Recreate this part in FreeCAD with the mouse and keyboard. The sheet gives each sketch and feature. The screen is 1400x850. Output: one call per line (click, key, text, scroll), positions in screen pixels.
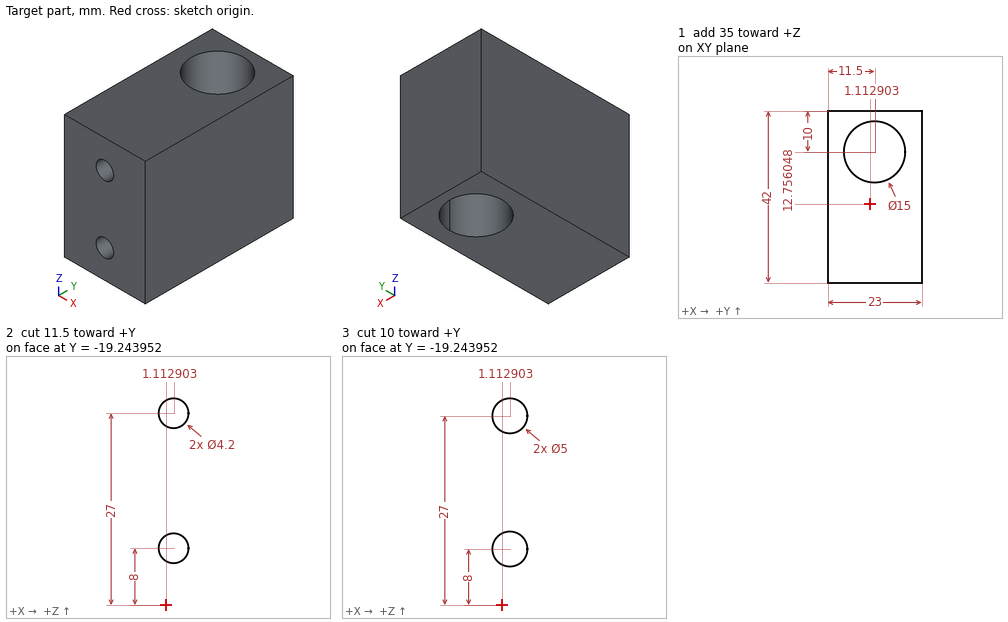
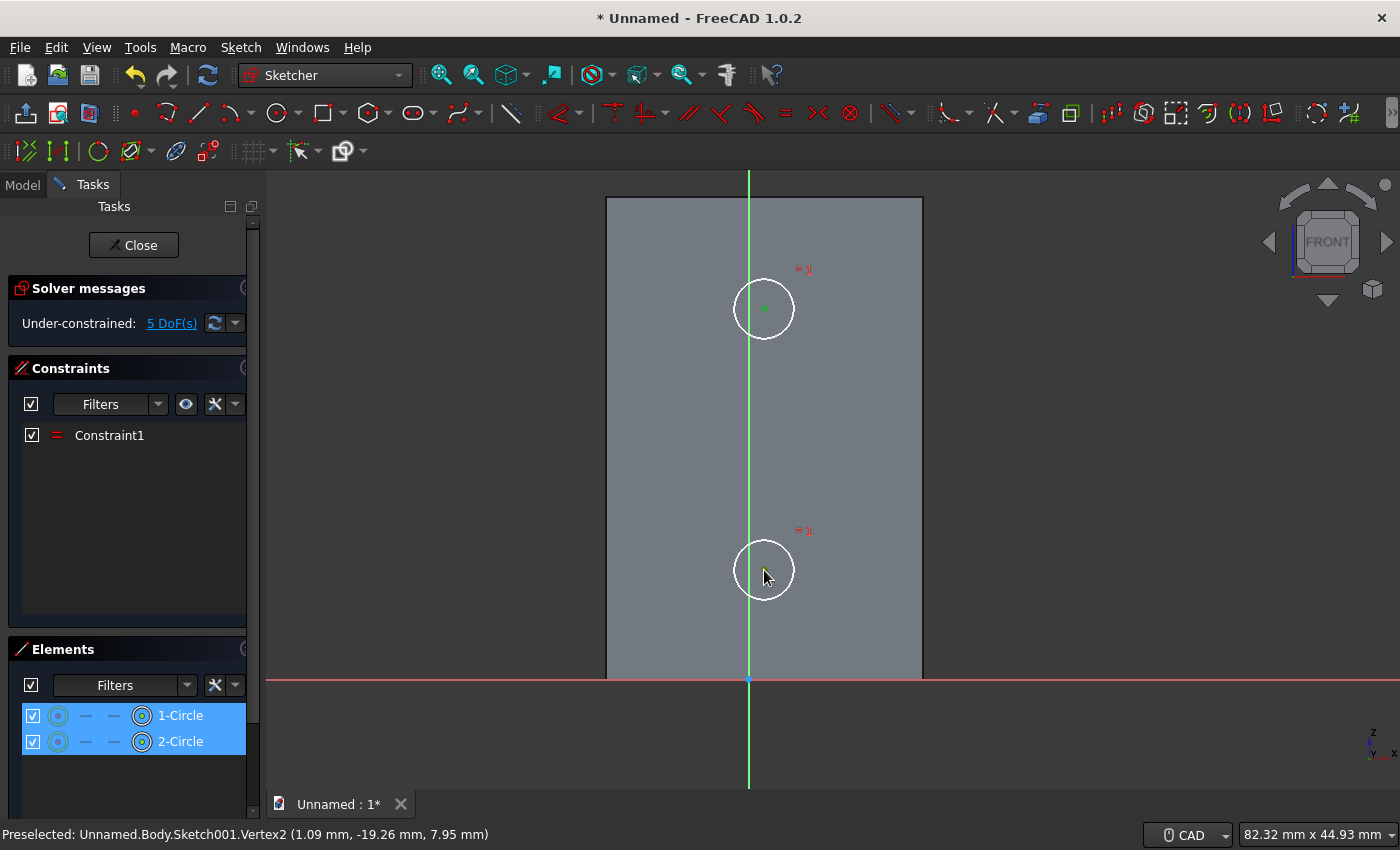
key(v)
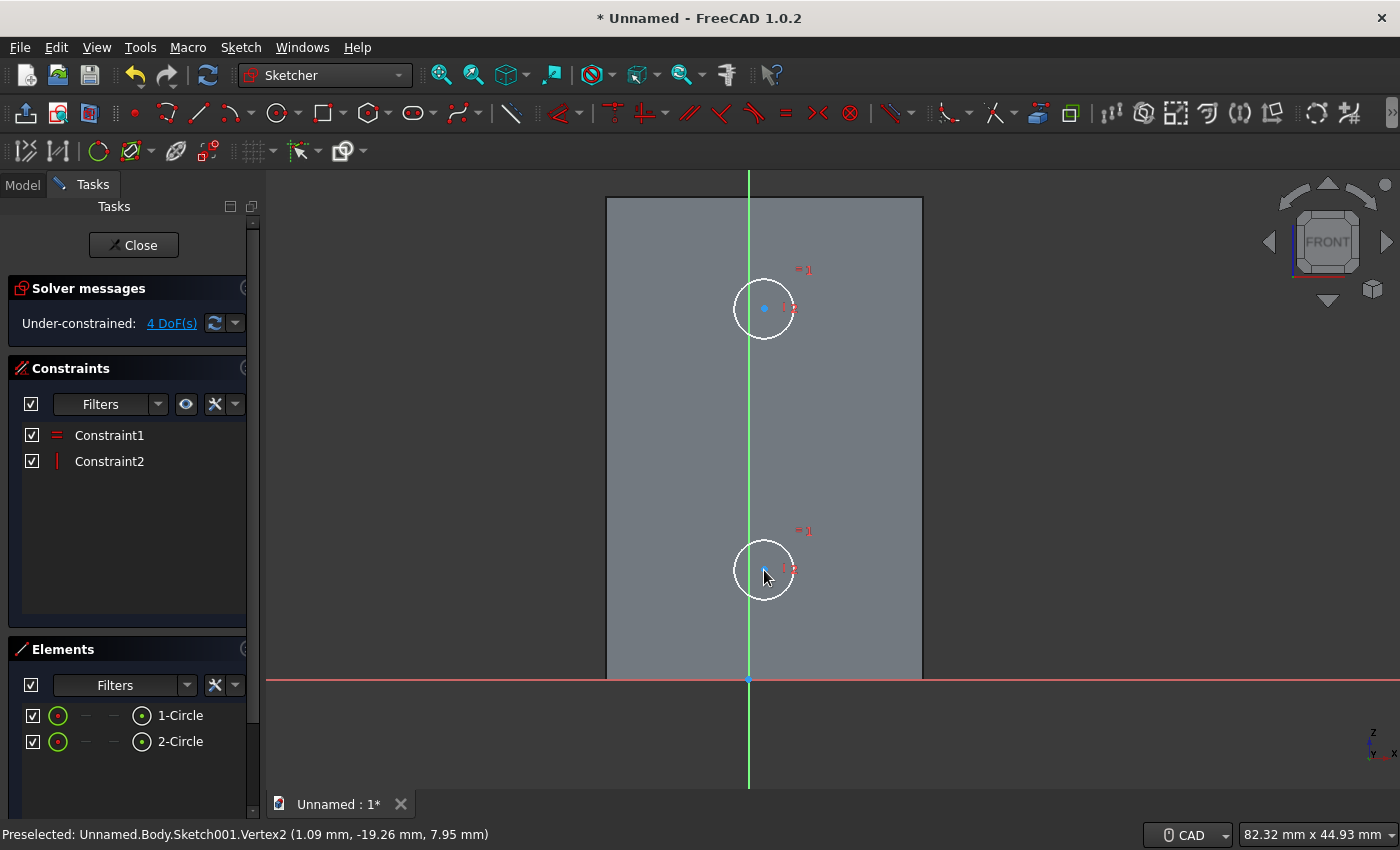
click(558, 114)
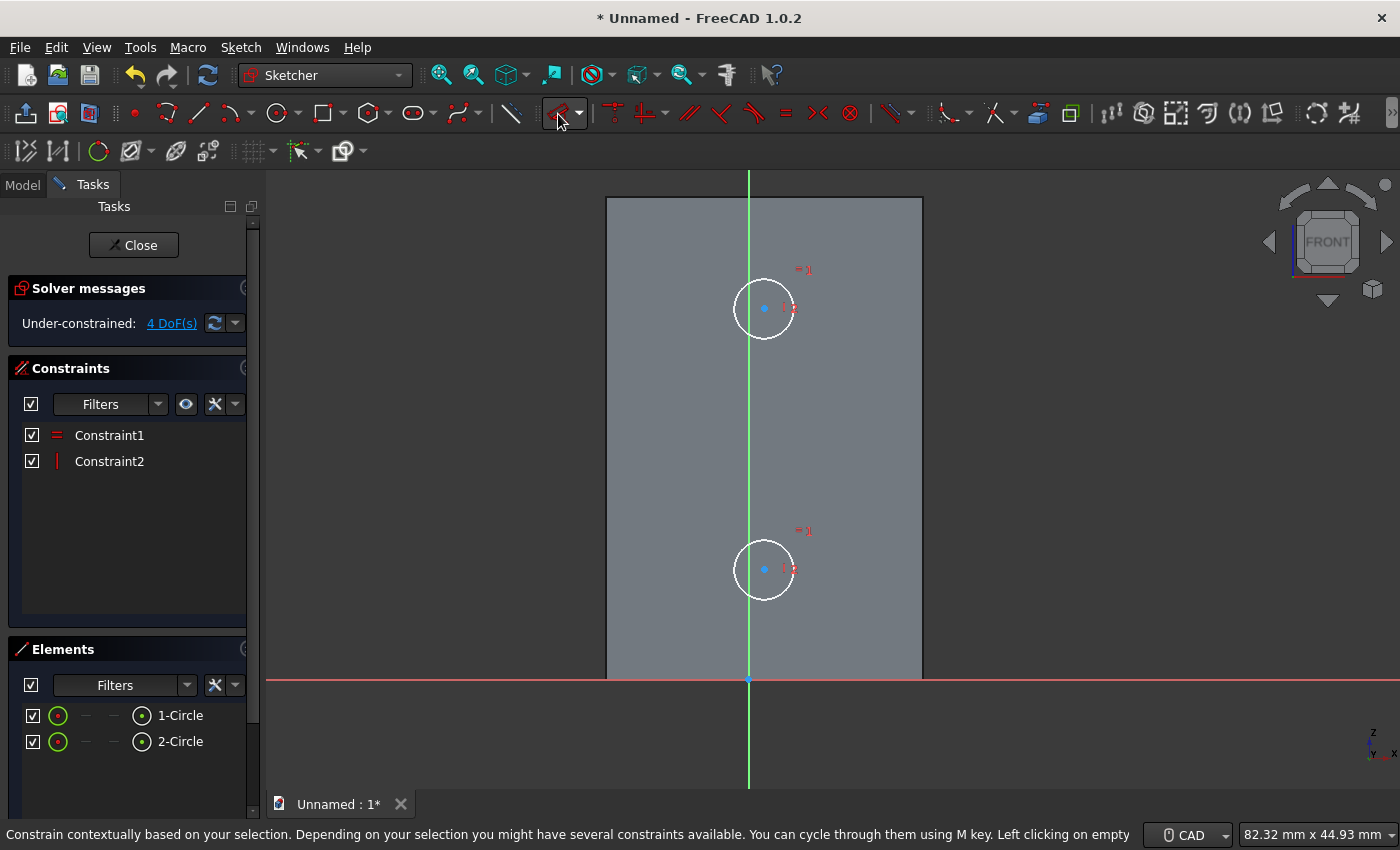
click(785, 288)
click(808, 265)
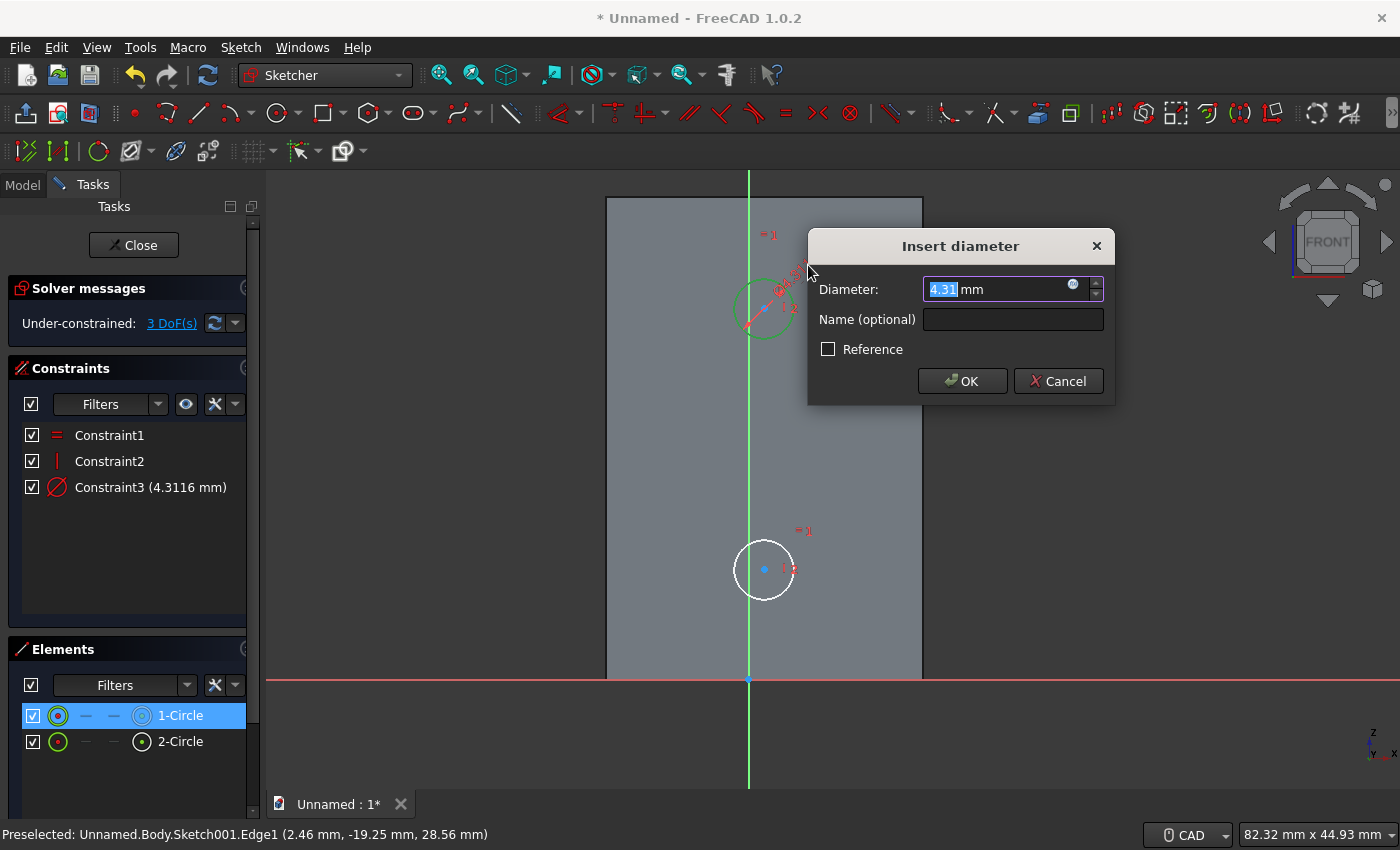
text(4.2)
key(Return)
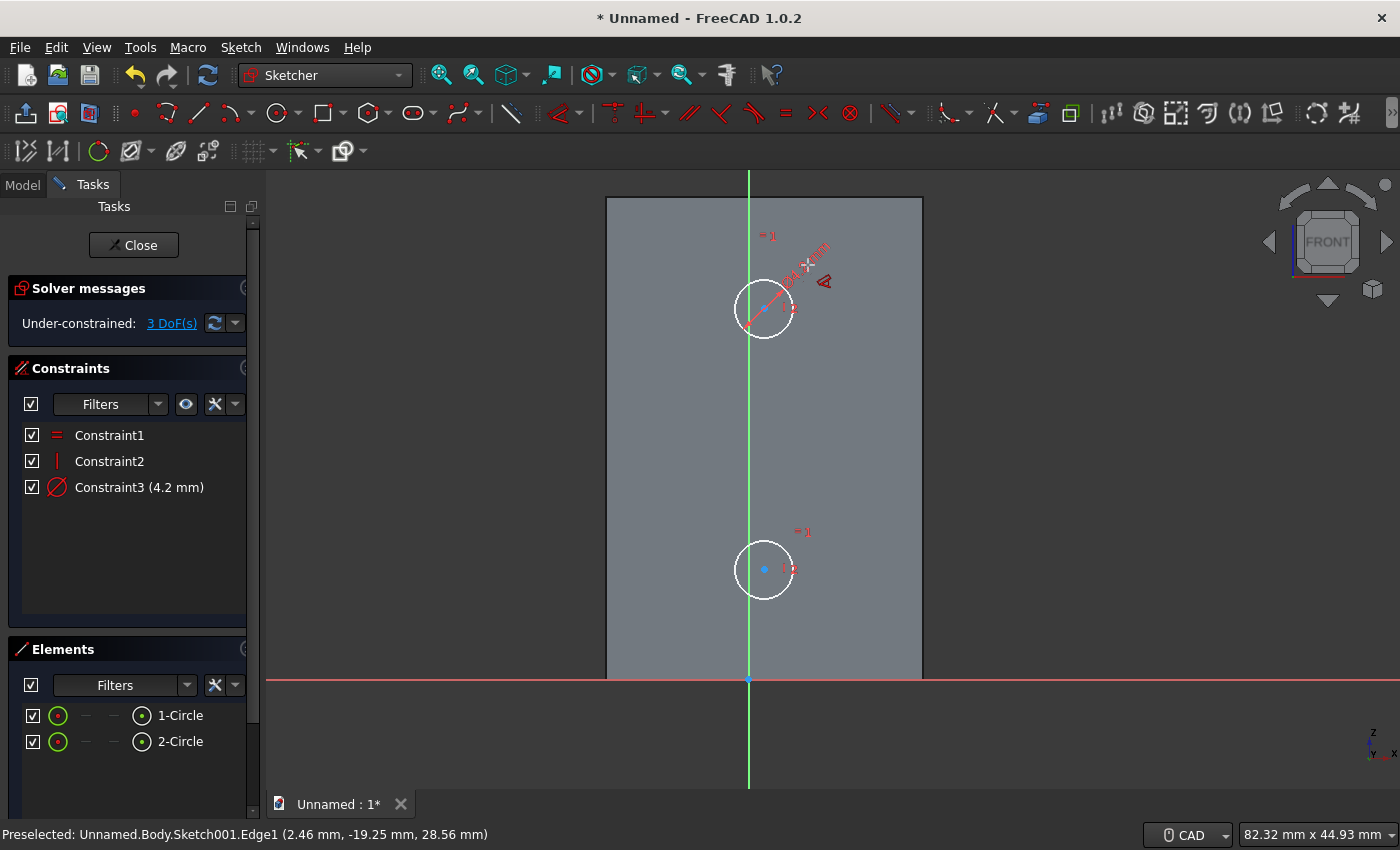
click(764, 570)
click(715, 625)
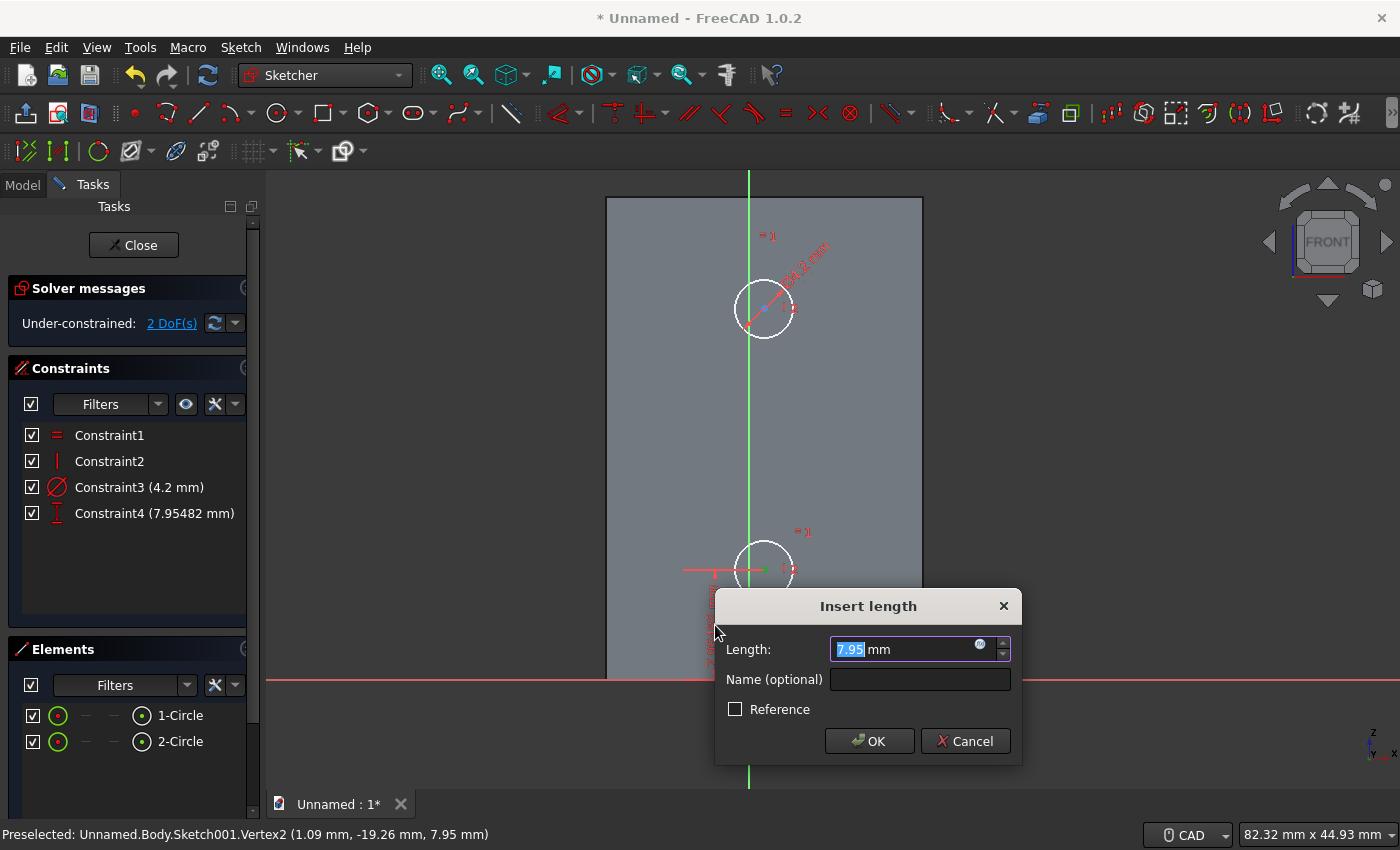
text(8)
key(Return)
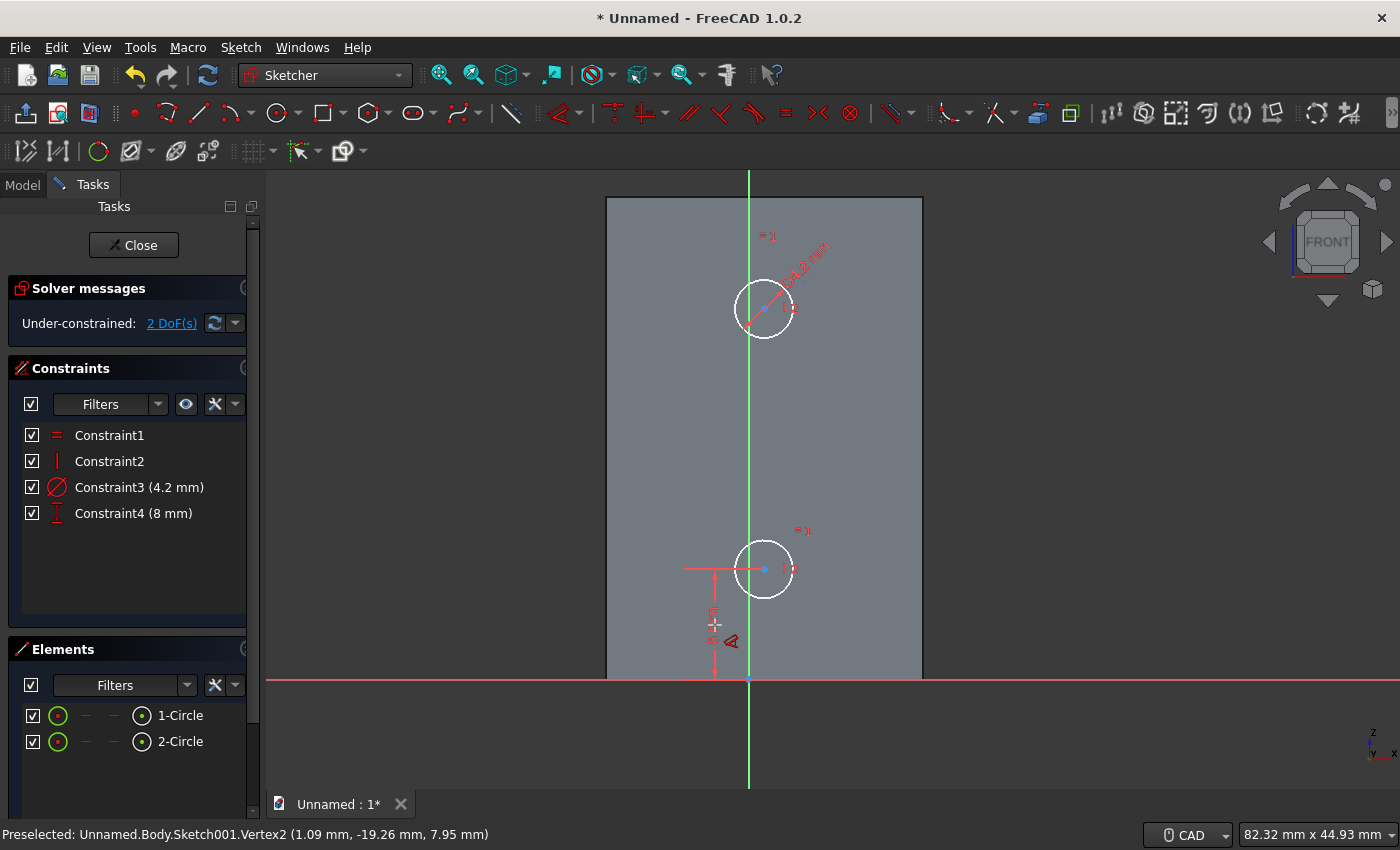
click(764, 309)
click(715, 494)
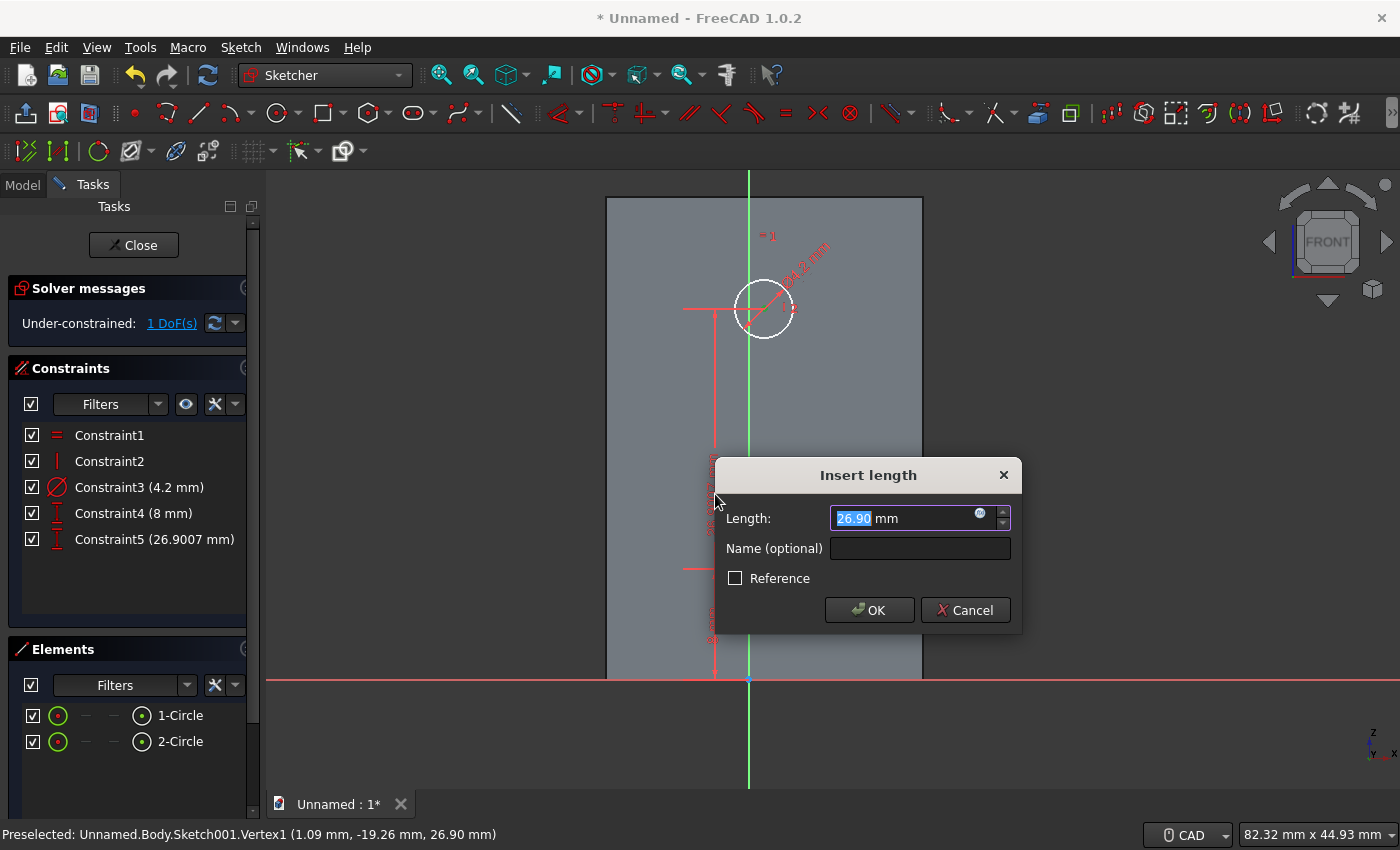
text(27)
key(Return)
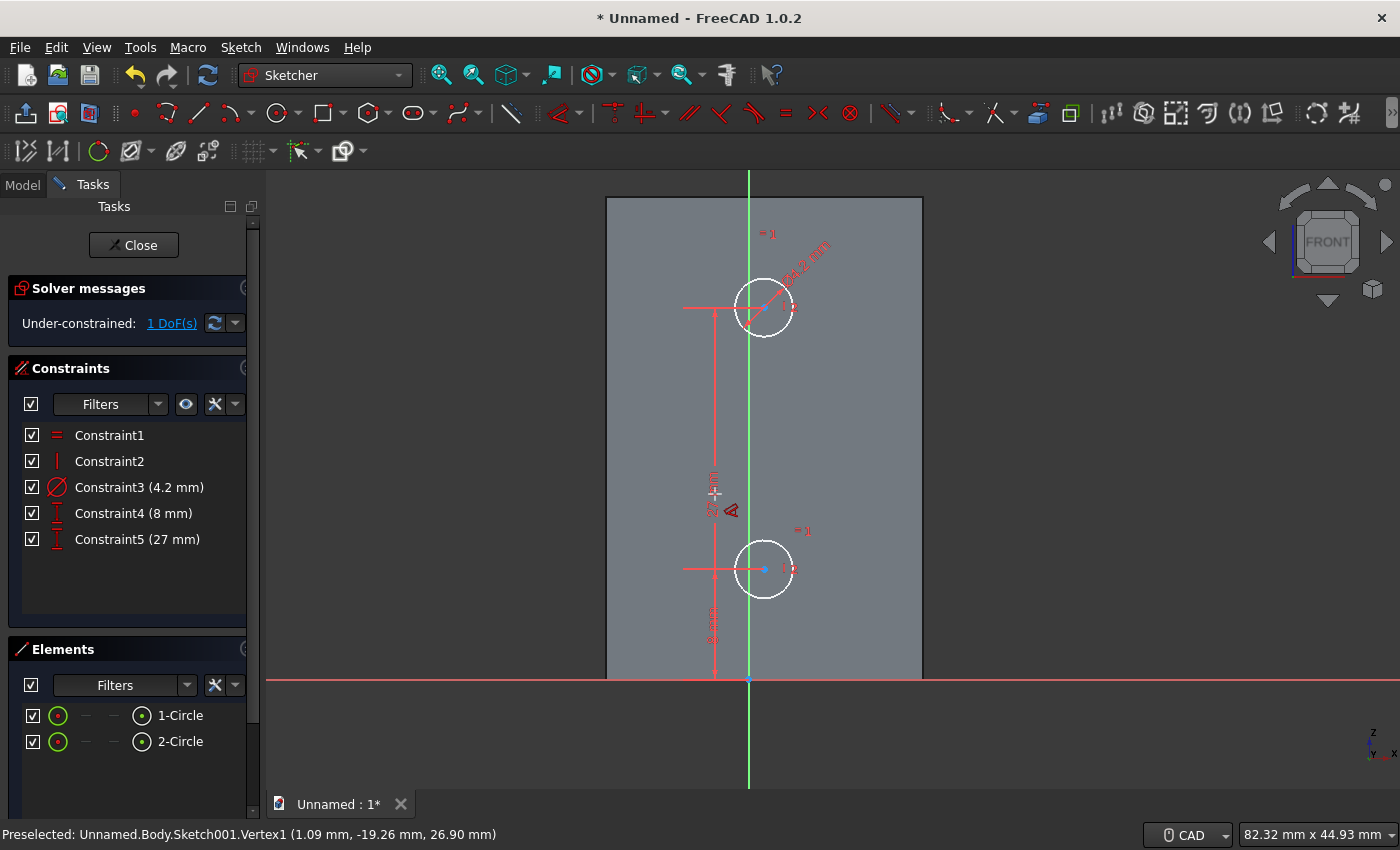
scroll(764, 308, up, 5)